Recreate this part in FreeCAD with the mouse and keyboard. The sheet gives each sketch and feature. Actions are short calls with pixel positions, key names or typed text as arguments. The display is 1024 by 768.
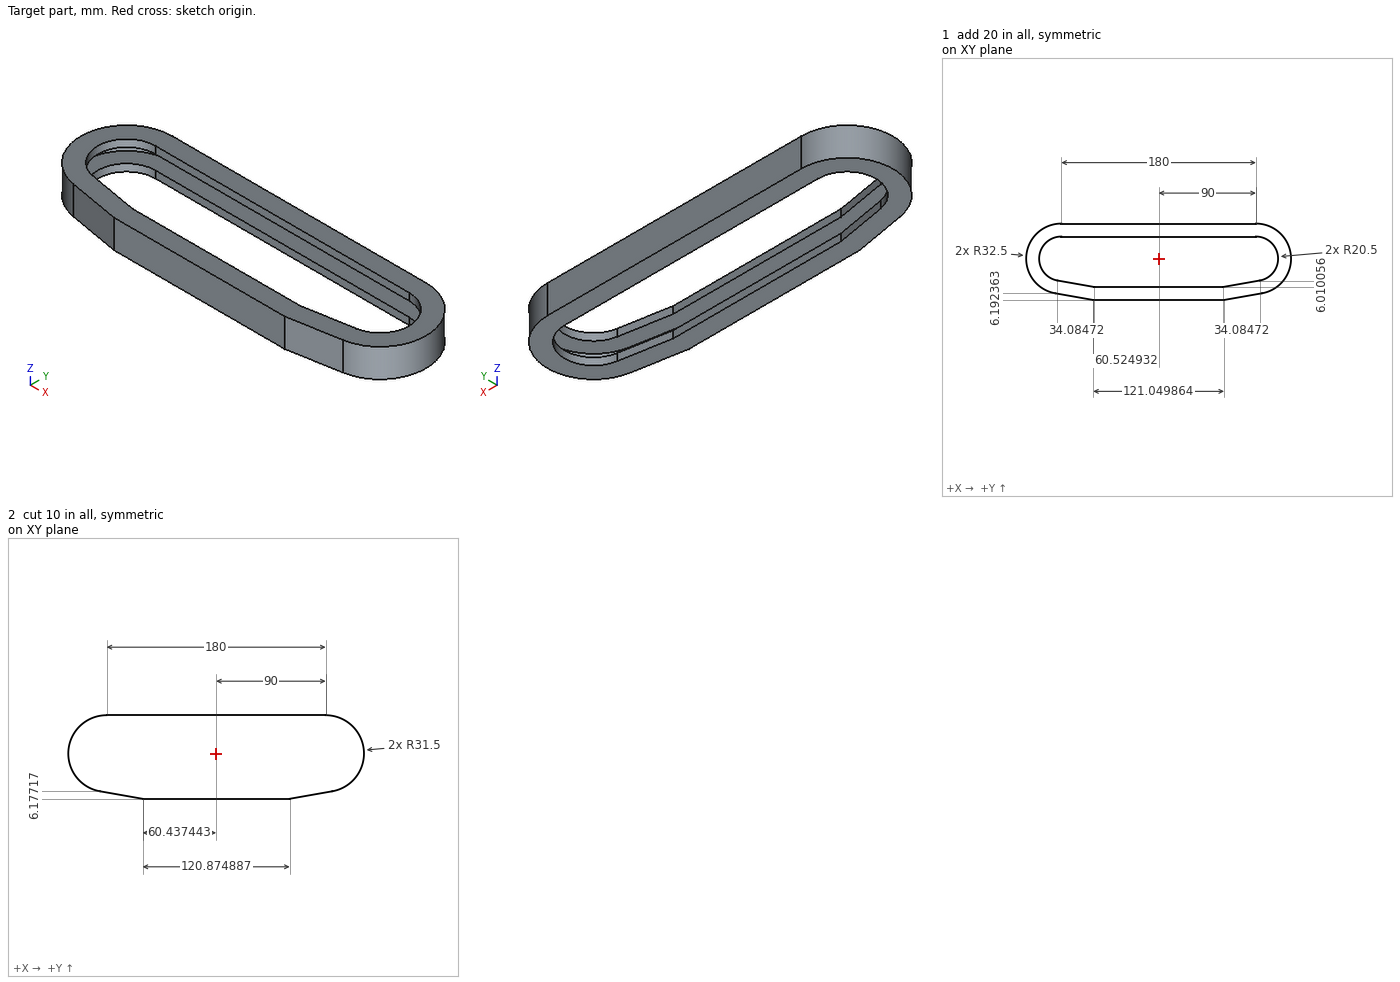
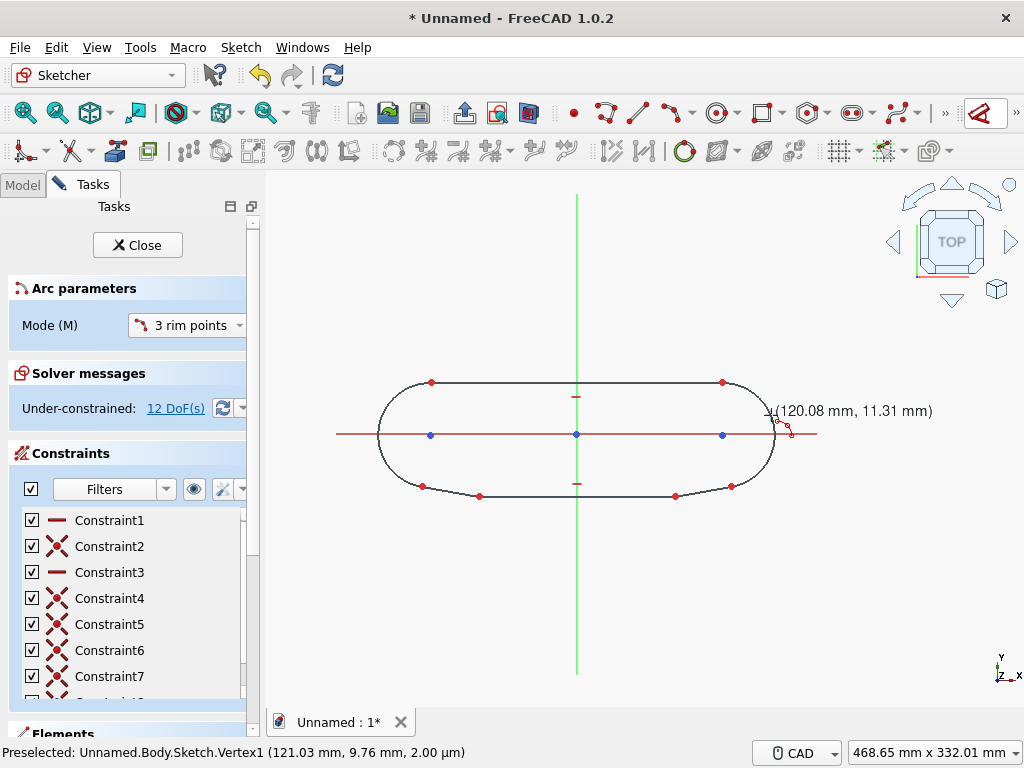
click(638, 114)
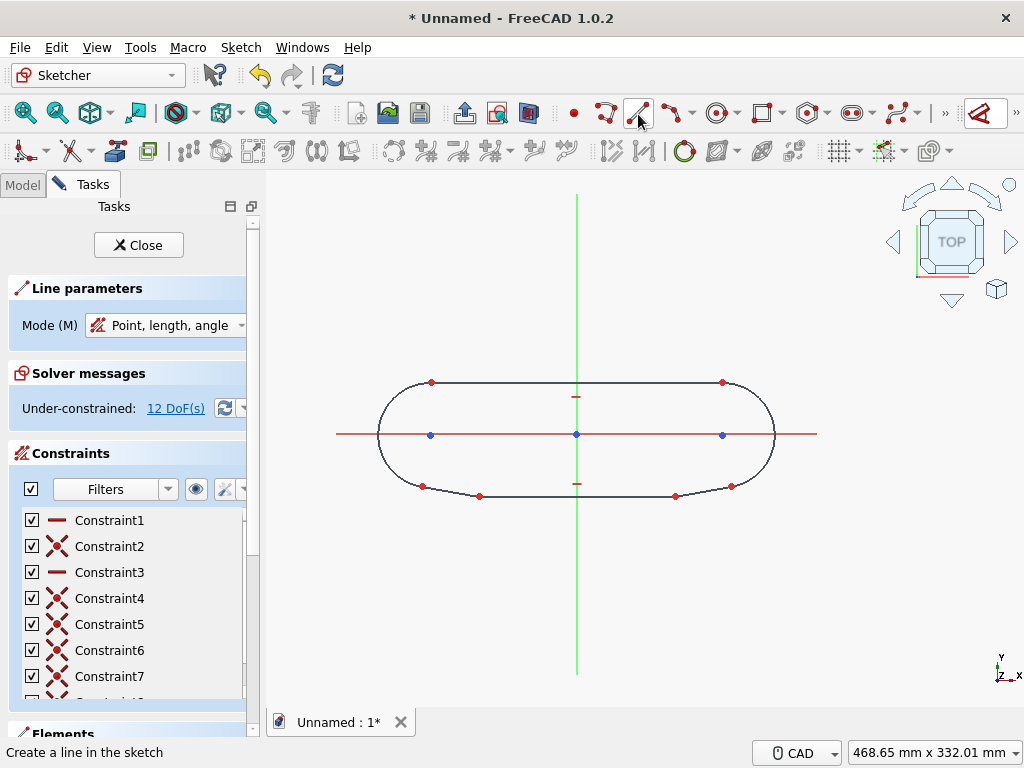
click(431, 401)
click(722, 401)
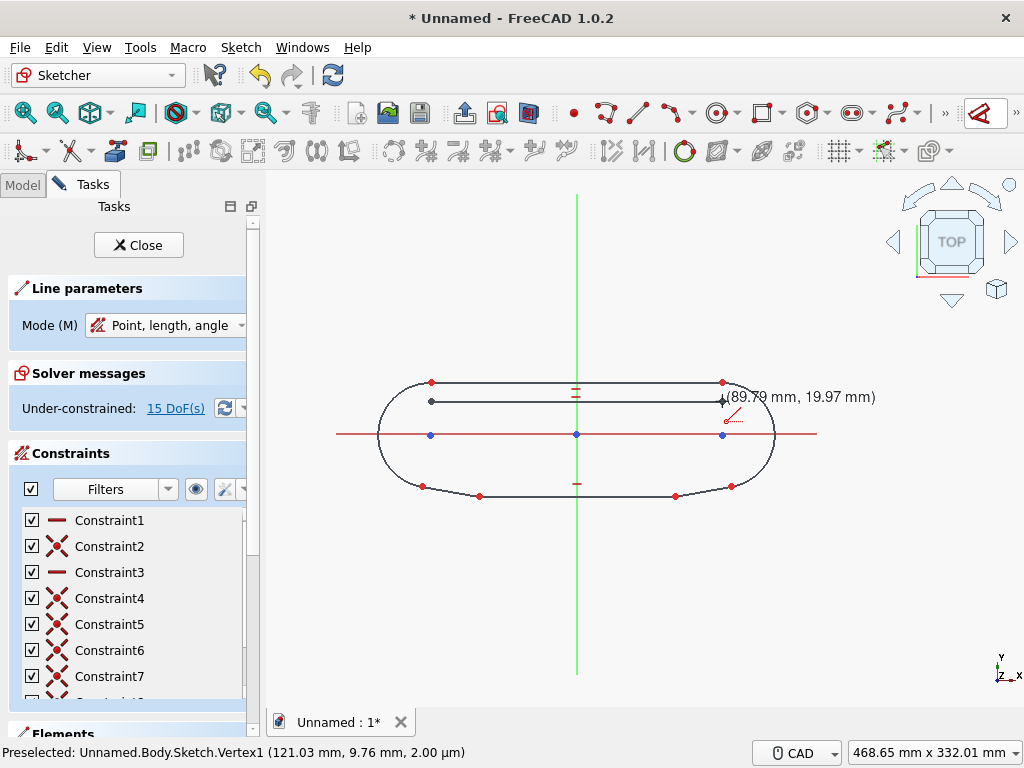
key(g)
key(m)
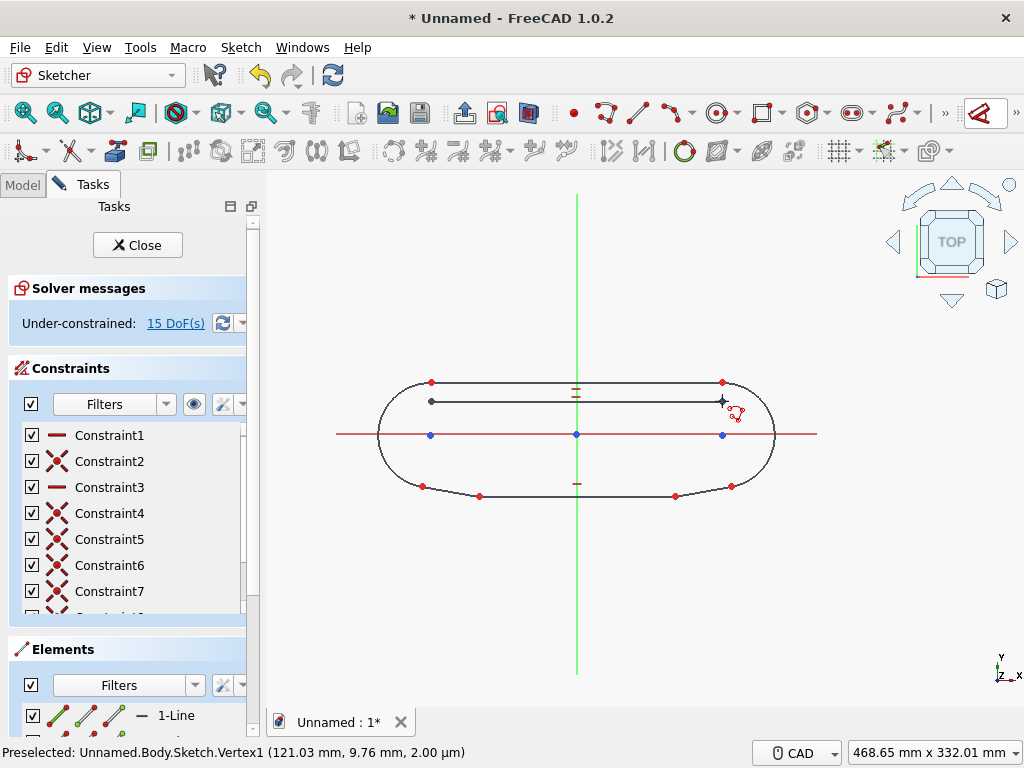
click(728, 467)
click(673, 477)
click(481, 477)
click(425, 467)
right_click(425, 467)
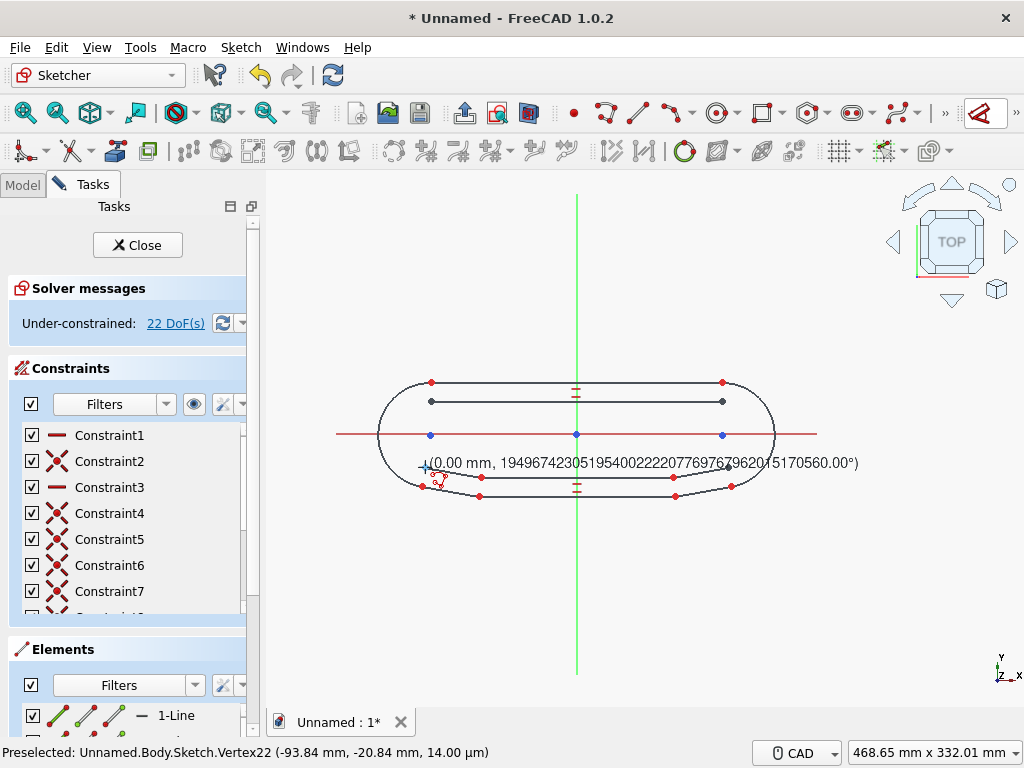
click(672, 114)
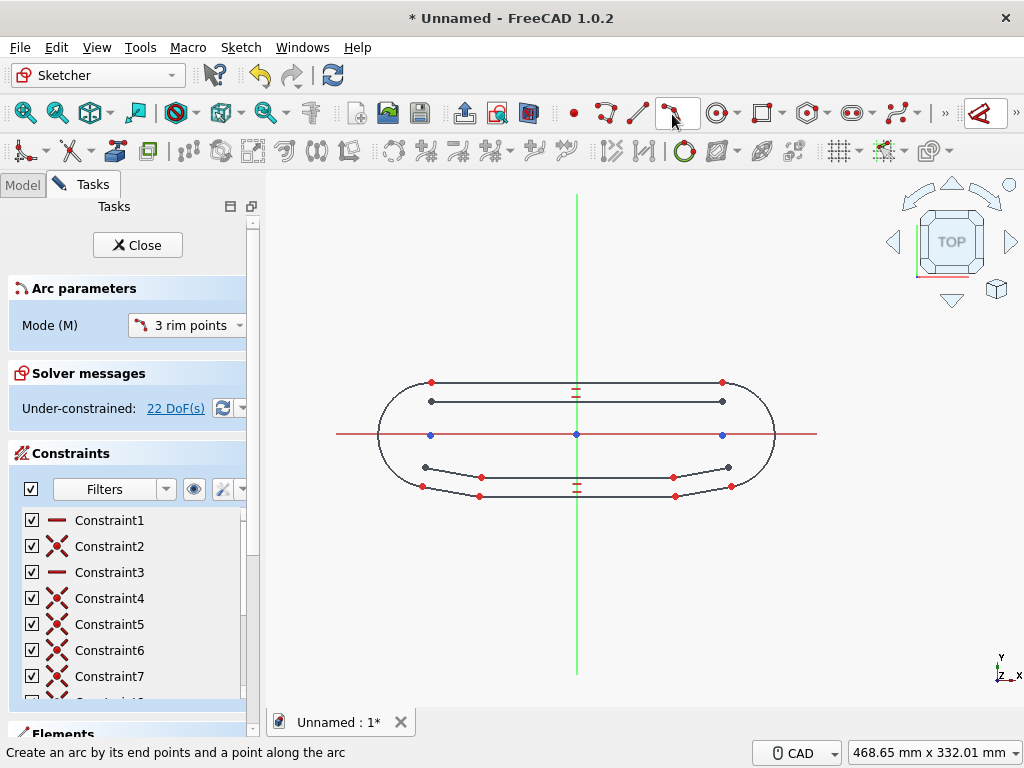
click(722, 402)
click(728, 468)
click(751, 450)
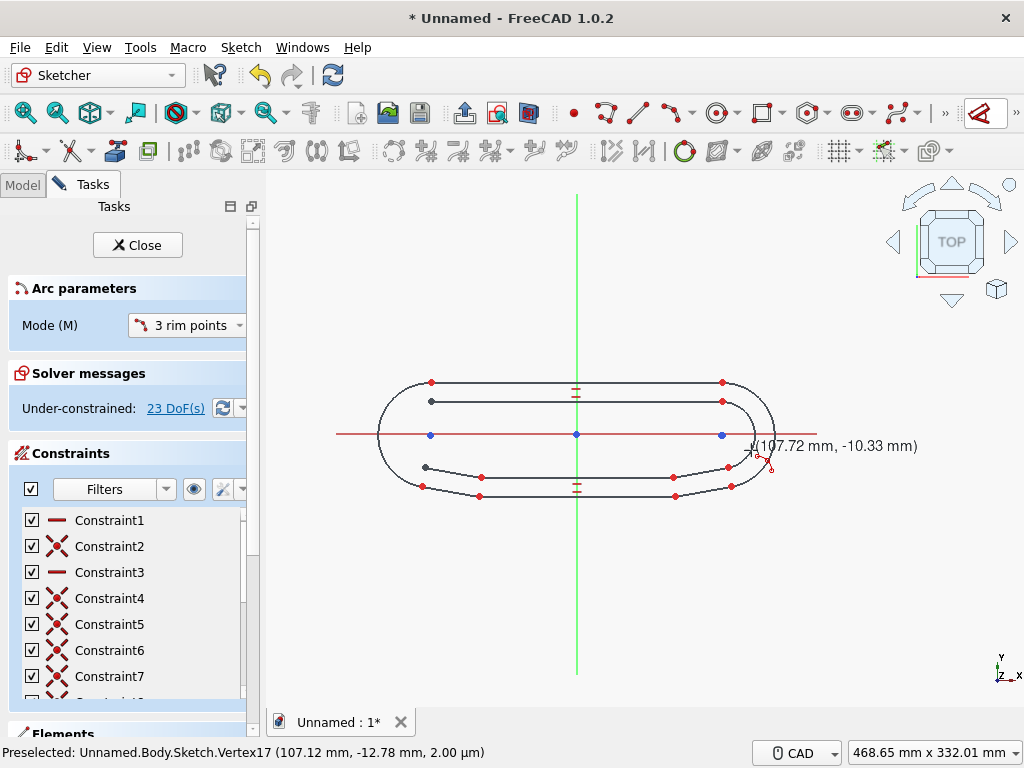
click(425, 468)
click(431, 402)
click(405, 413)
key(Escape)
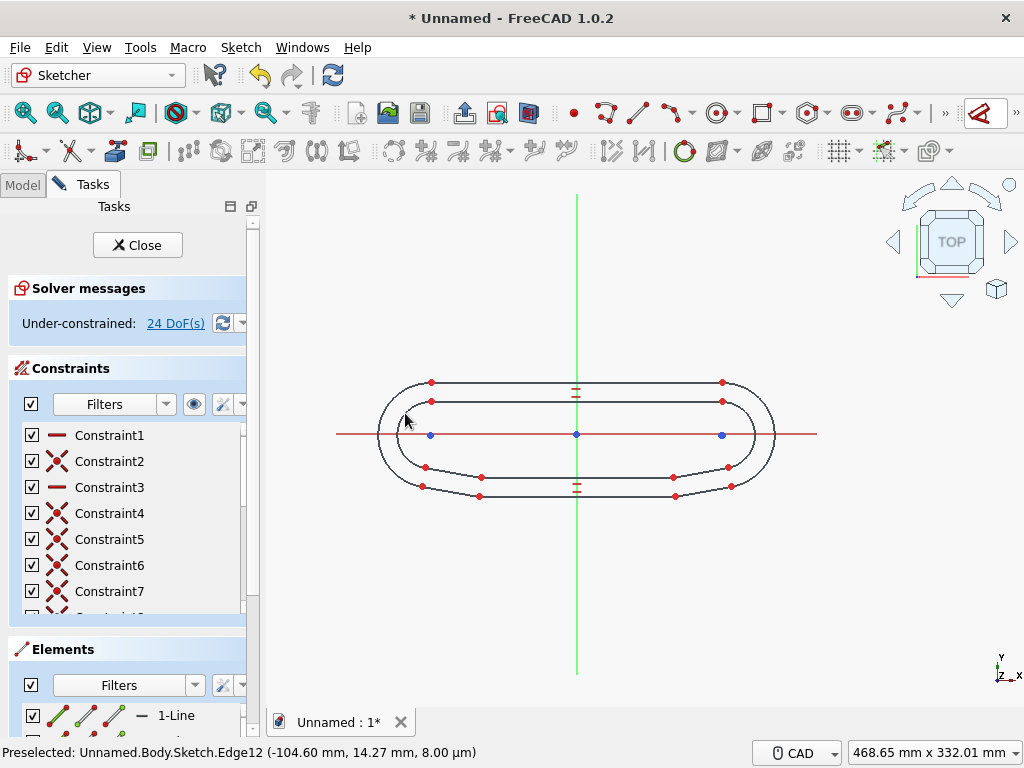
click(635, 383)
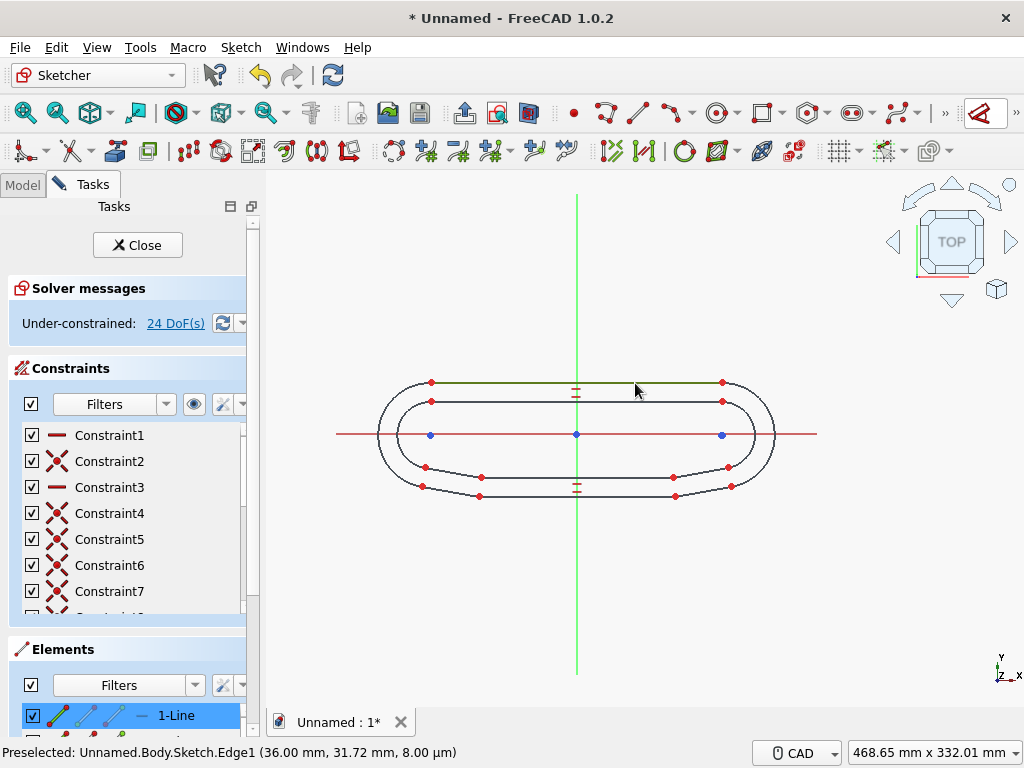
click(390, 402)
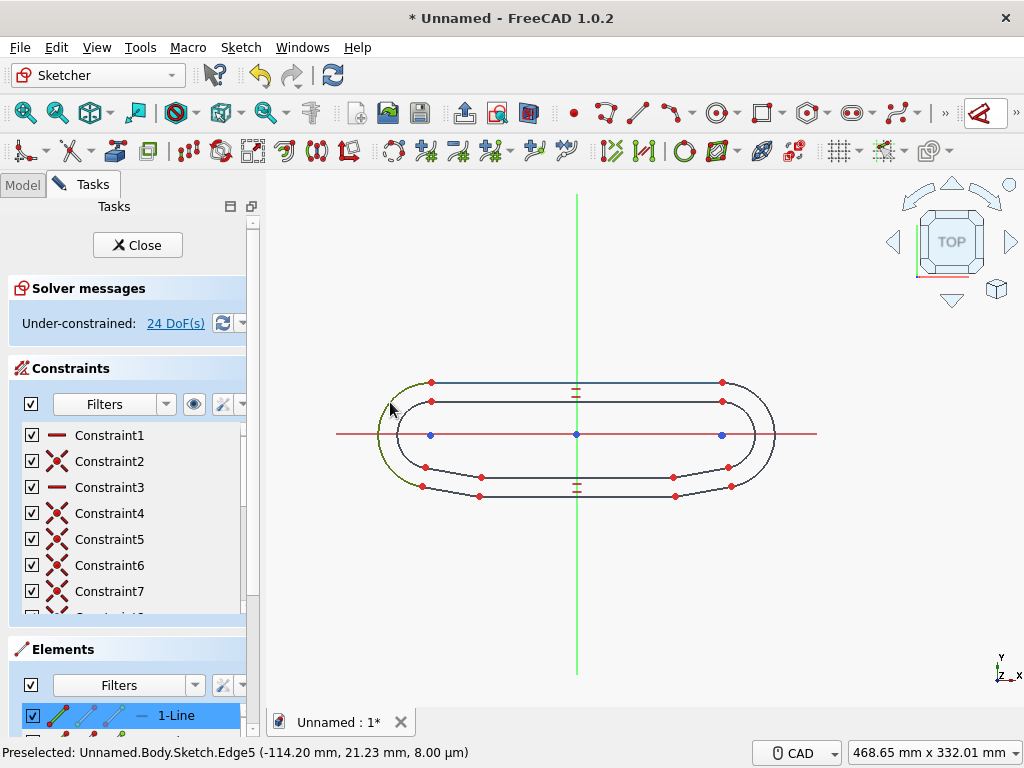
key(t)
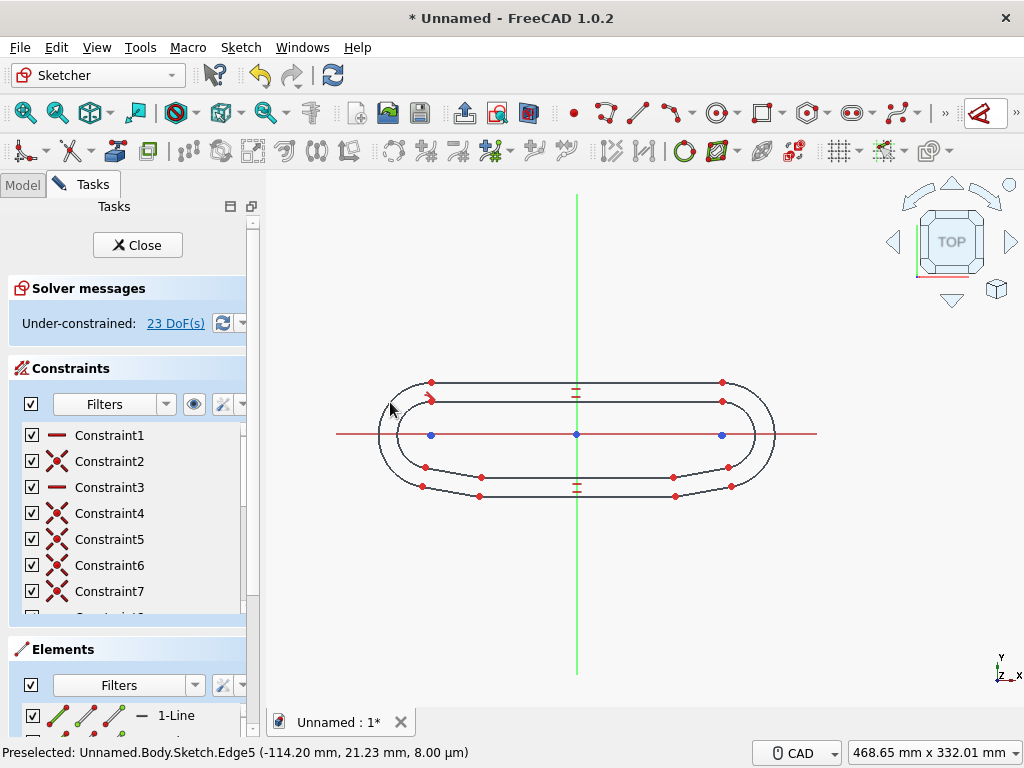
click(635, 383)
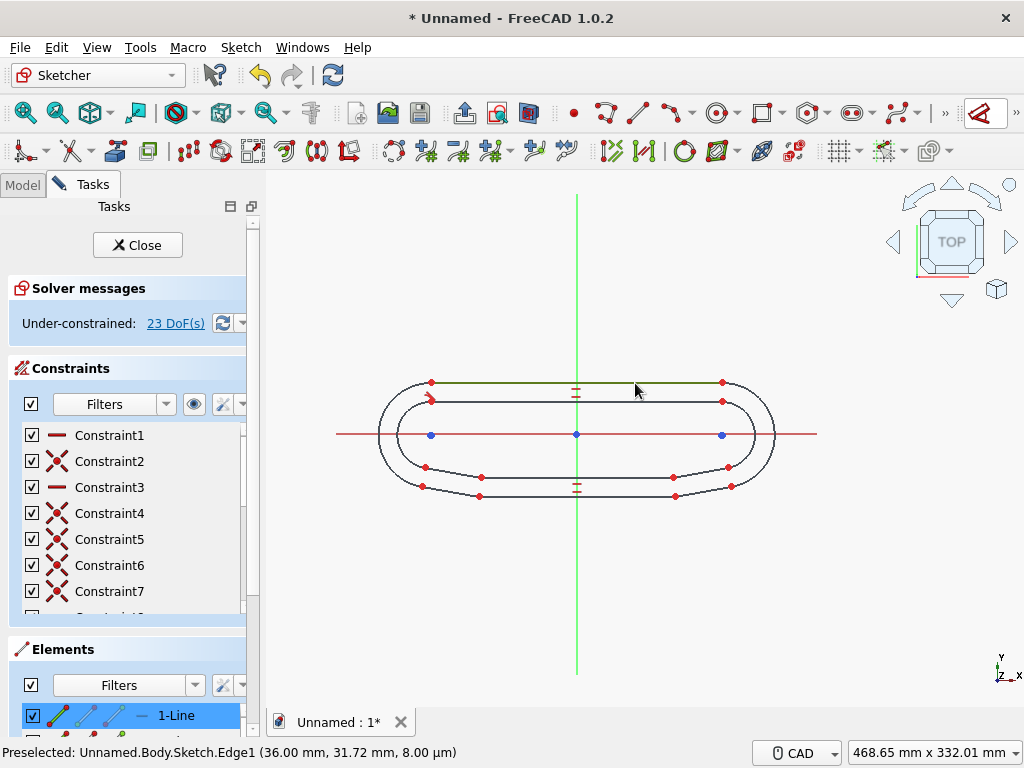
click(768, 461)